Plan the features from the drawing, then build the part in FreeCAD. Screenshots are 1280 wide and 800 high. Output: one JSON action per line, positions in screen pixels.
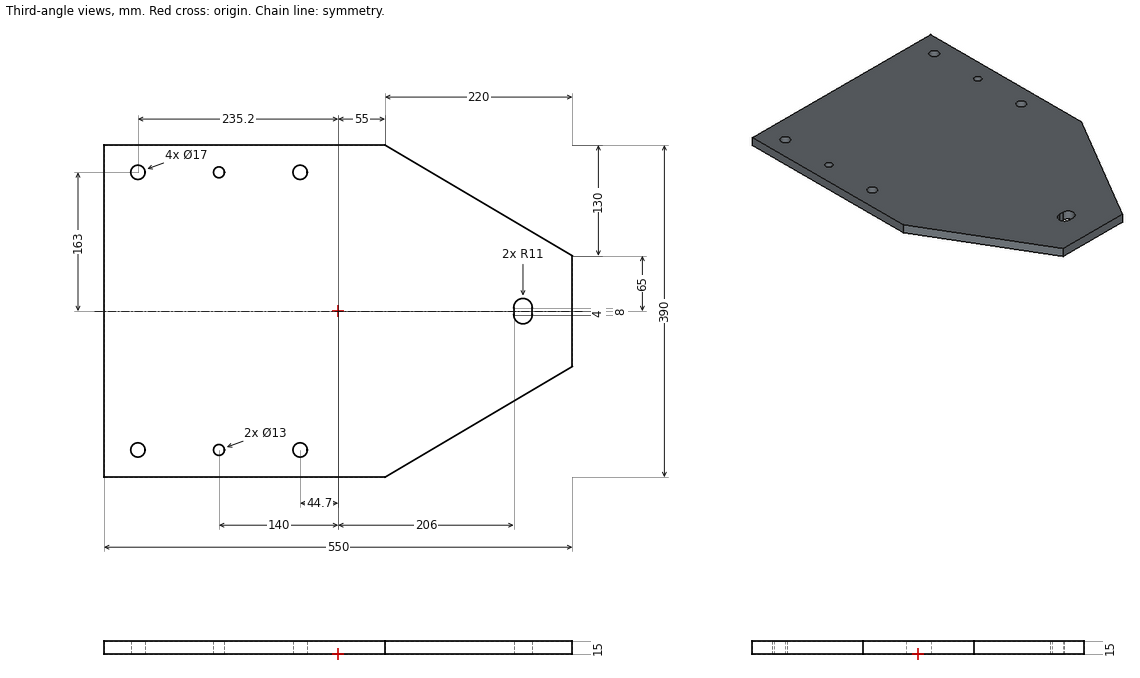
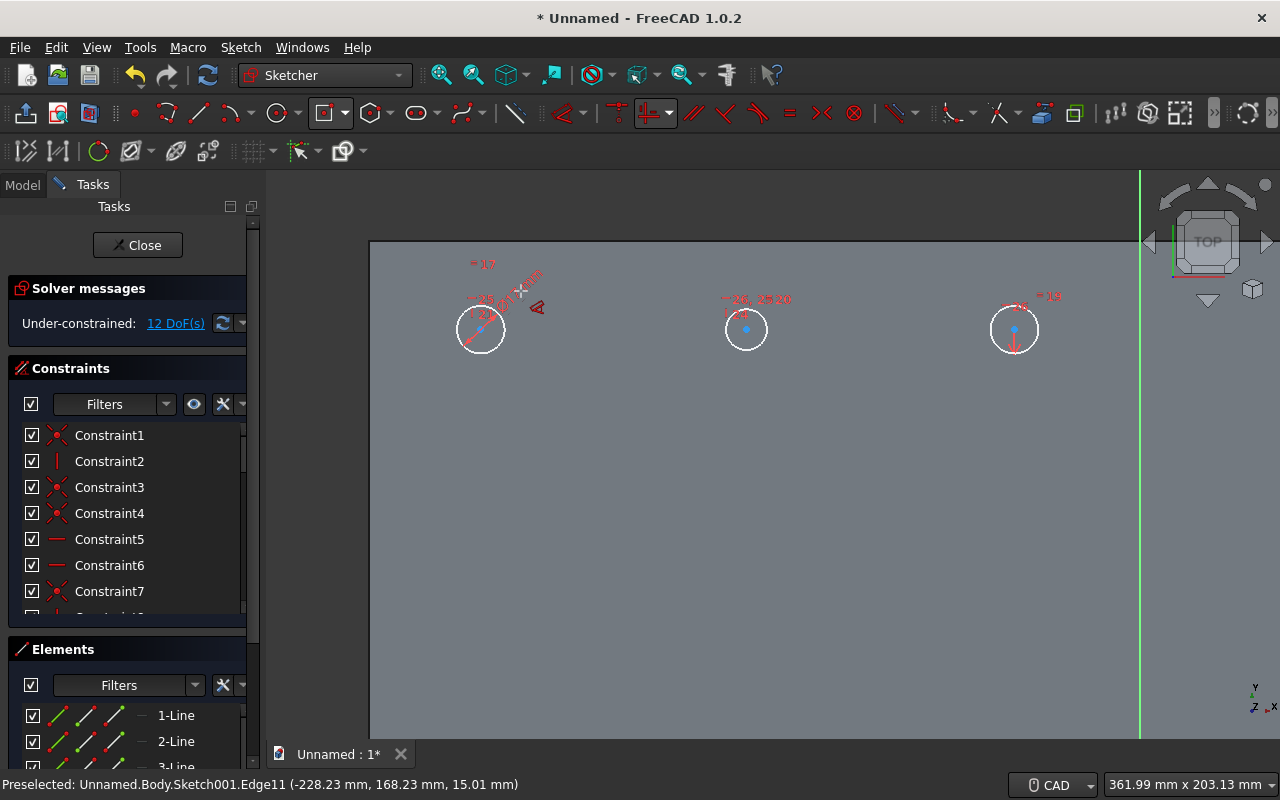
{"action": "scroll", "coordinate": [498, 311], "scroll_direction": "down", "scroll_amount": 6}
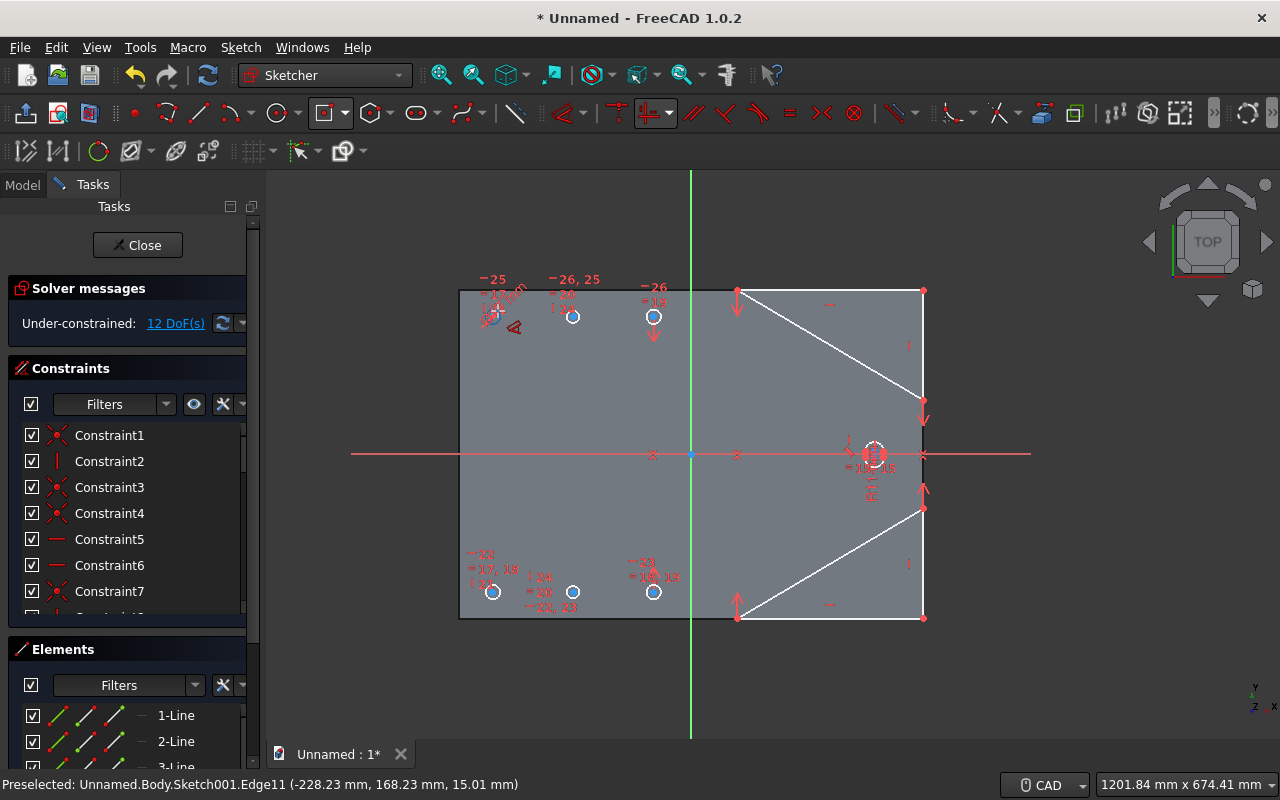
{"action": "scroll", "coordinate": [577, 588], "scroll_direction": "up", "scroll_amount": 7}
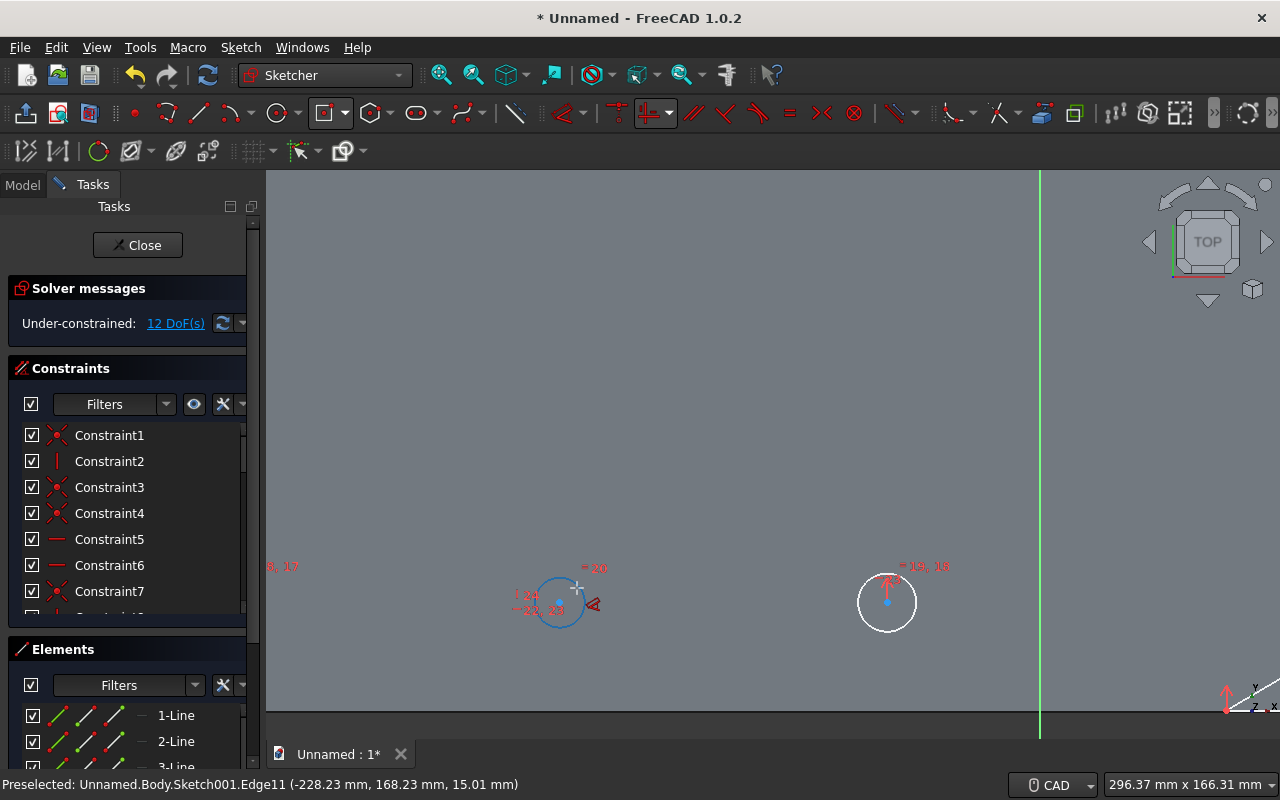
{"action": "left_click", "coordinate": [577, 585]}
{"action": "left_click", "coordinate": [599, 562]}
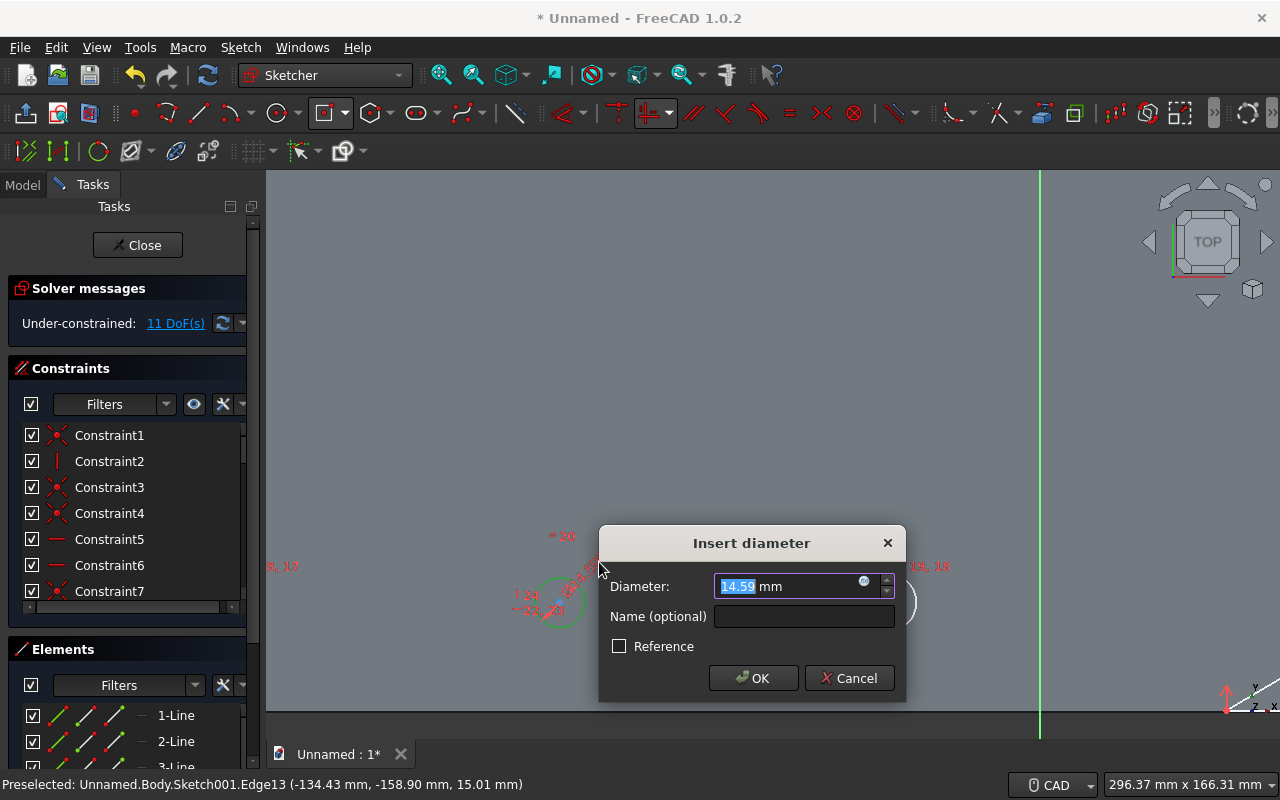
{"action": "type", "text": "13"}
{"action": "key", "text": "Return"}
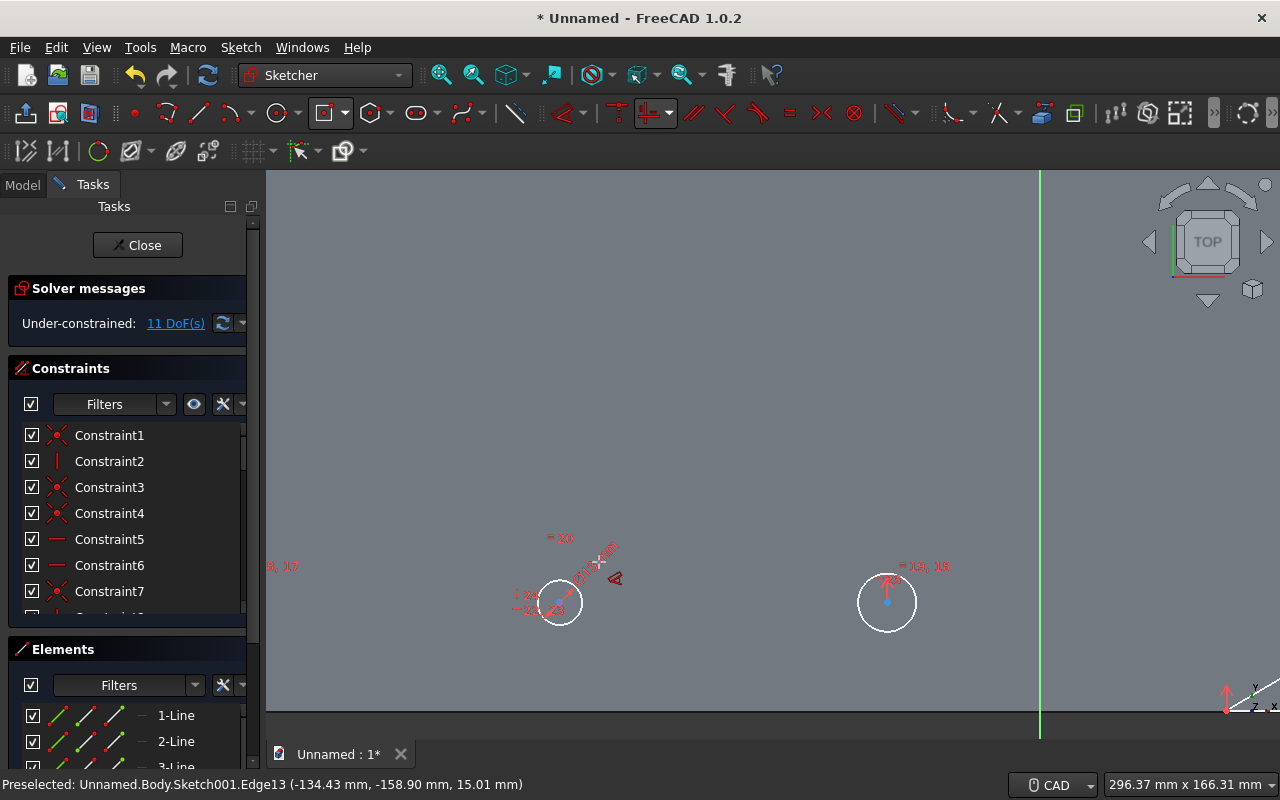
{"action": "scroll", "coordinate": [577, 589], "scroll_direction": "down", "scroll_amount": 7}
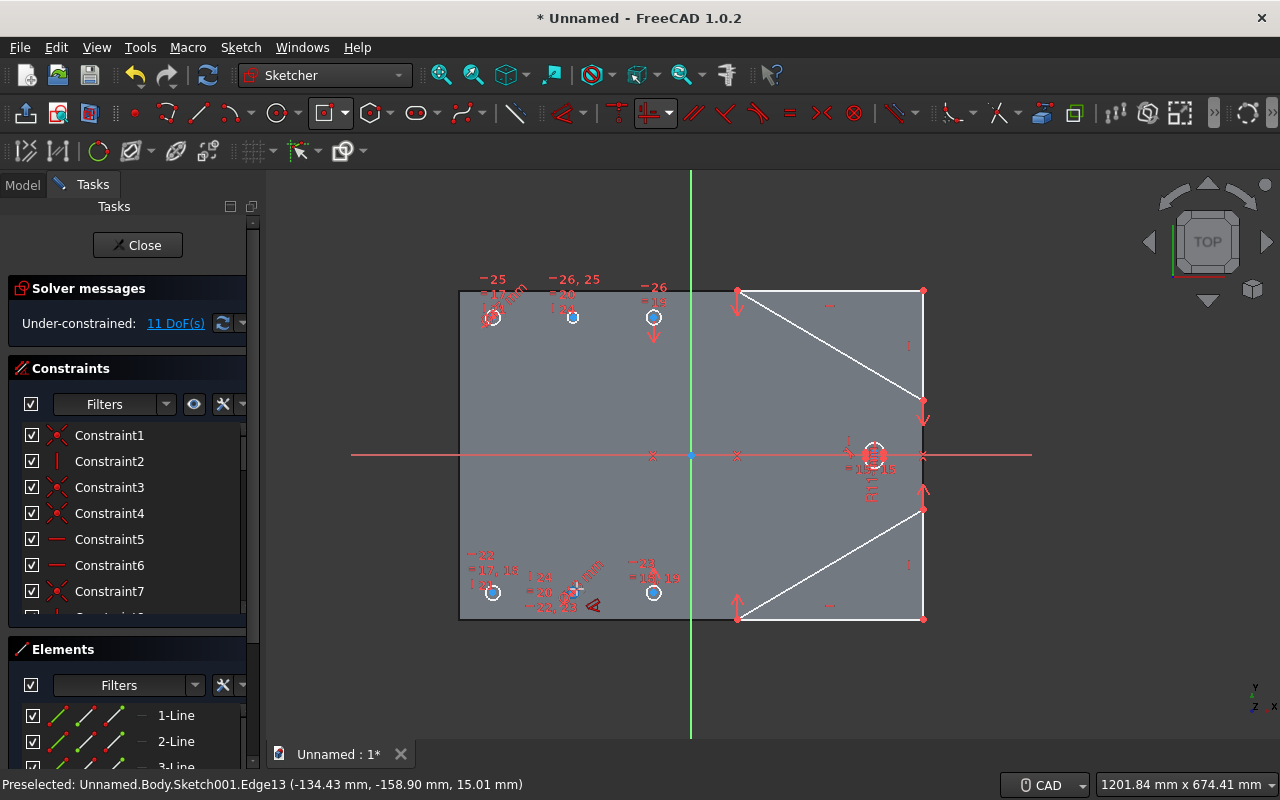
{"action": "scroll", "coordinate": [865, 456], "scroll_direction": "up", "scroll_amount": 9}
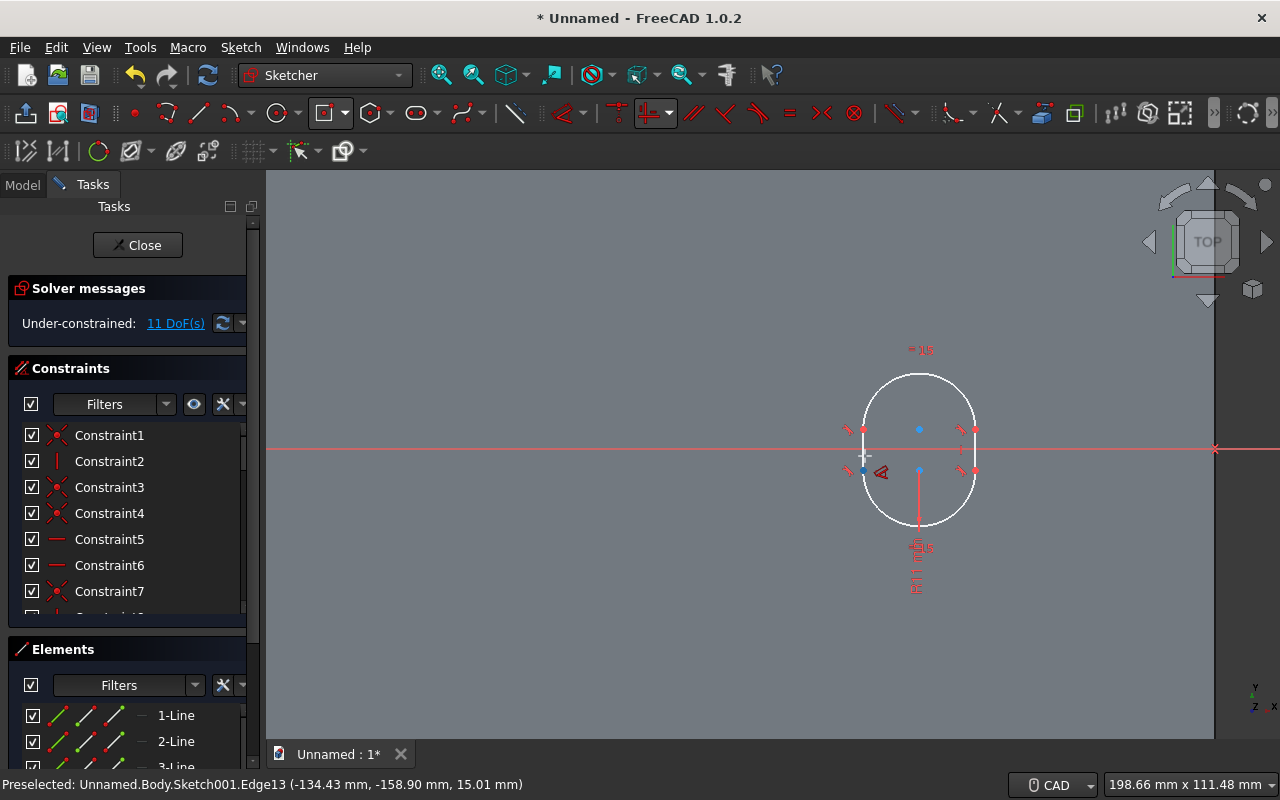
{"action": "left_click", "coordinate": [863, 454]}
{"action": "left_click", "coordinate": [897, 436]}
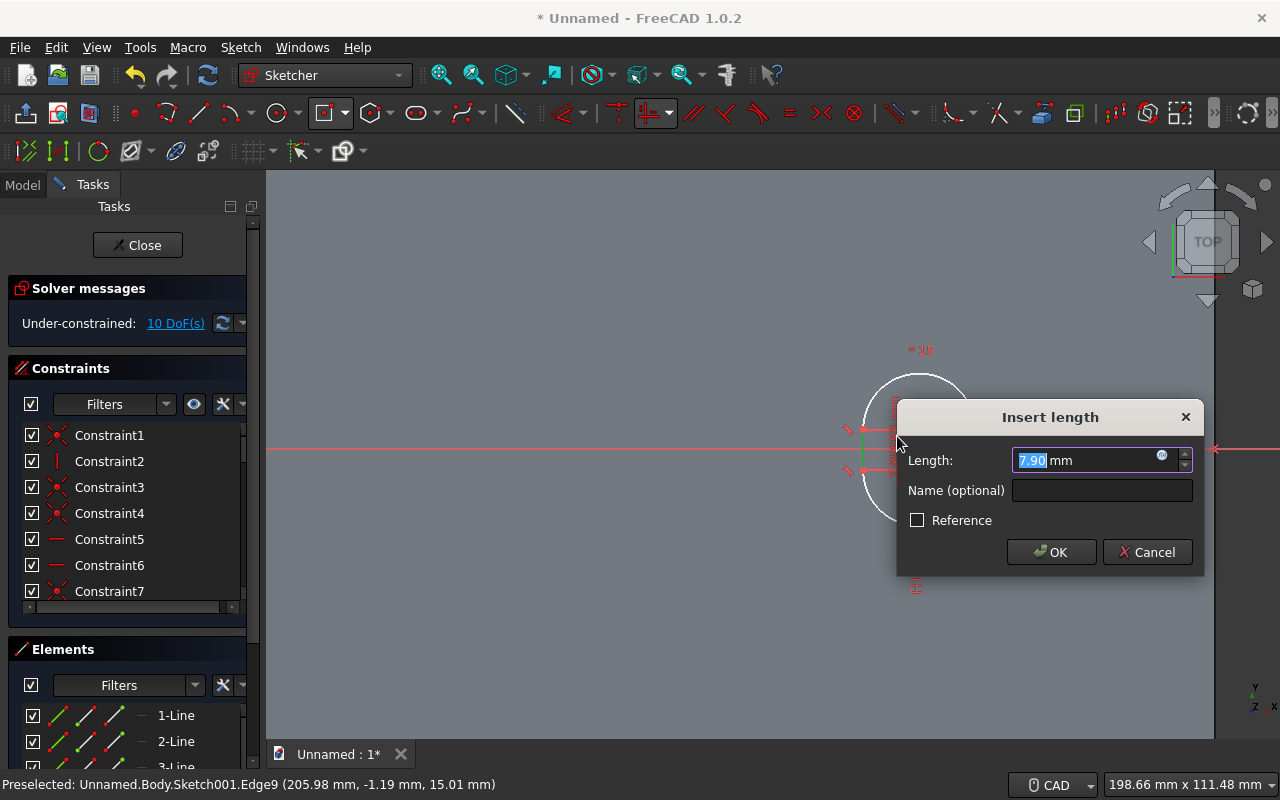
{"action": "type", "text": "8"}
{"action": "key", "text": "Return"}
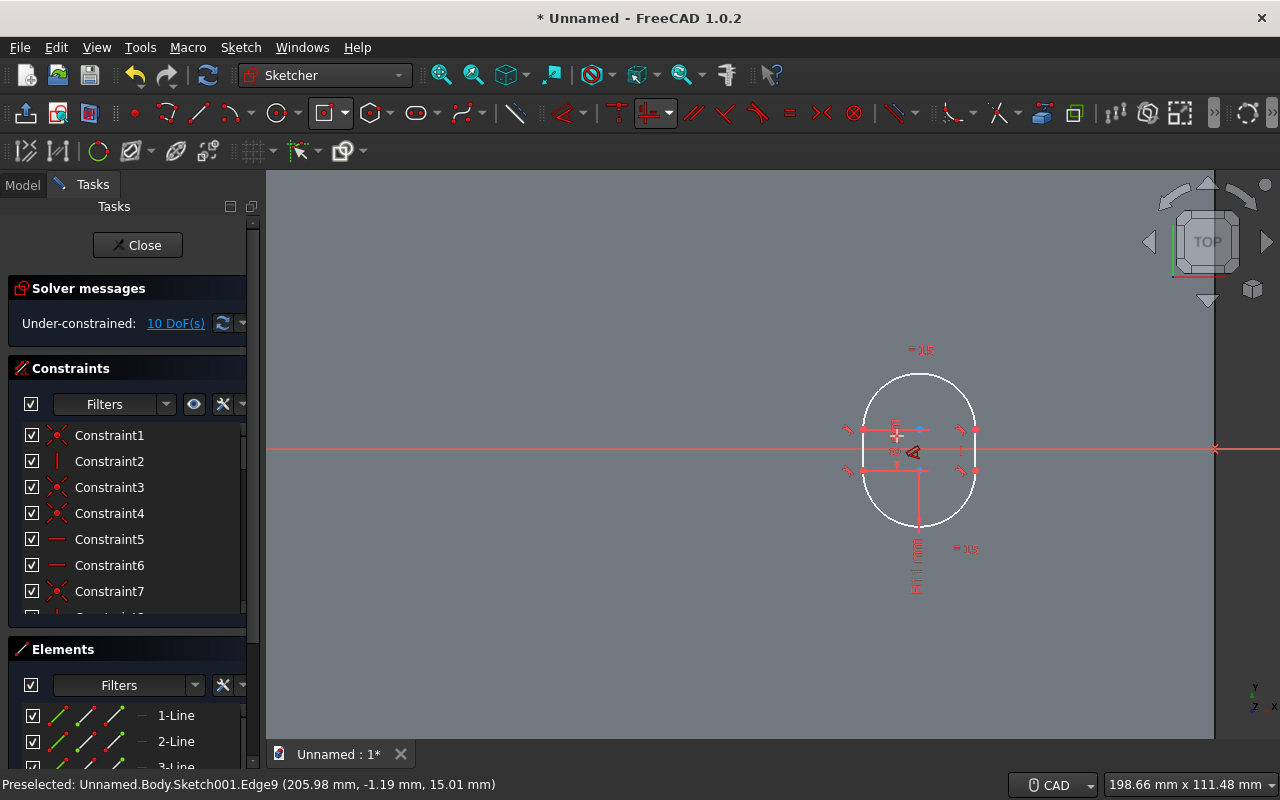
{"action": "scroll", "coordinate": [863, 471], "scroll_direction": "up", "scroll_amount": 4}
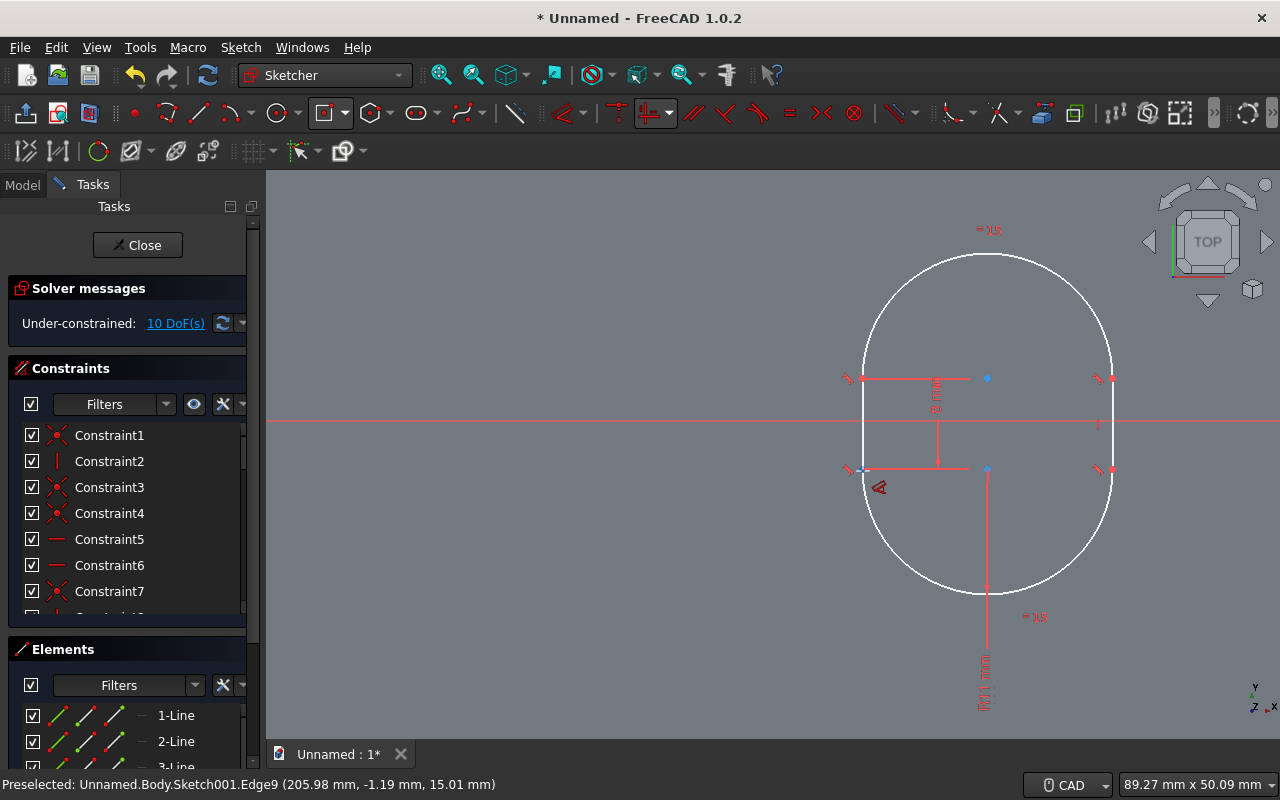
{"action": "left_click", "coordinate": [863, 469]}
{"action": "left_click", "coordinate": [897, 445]}